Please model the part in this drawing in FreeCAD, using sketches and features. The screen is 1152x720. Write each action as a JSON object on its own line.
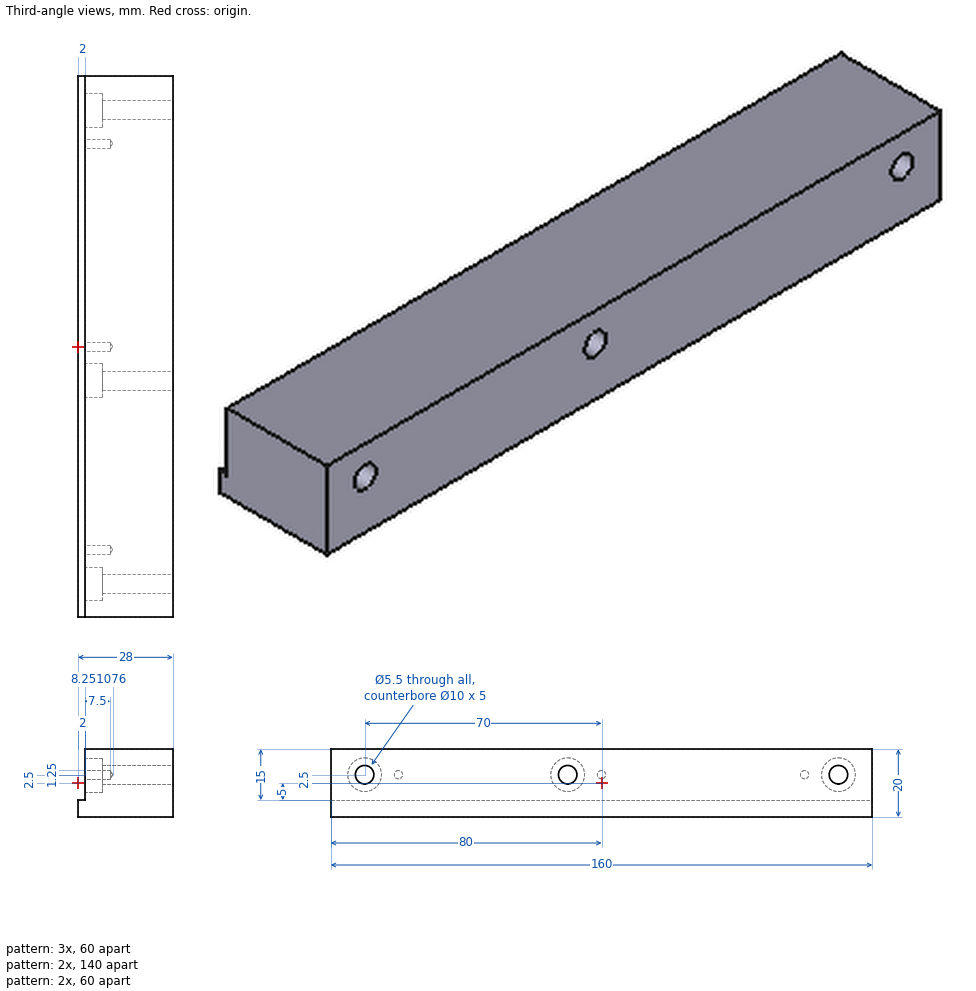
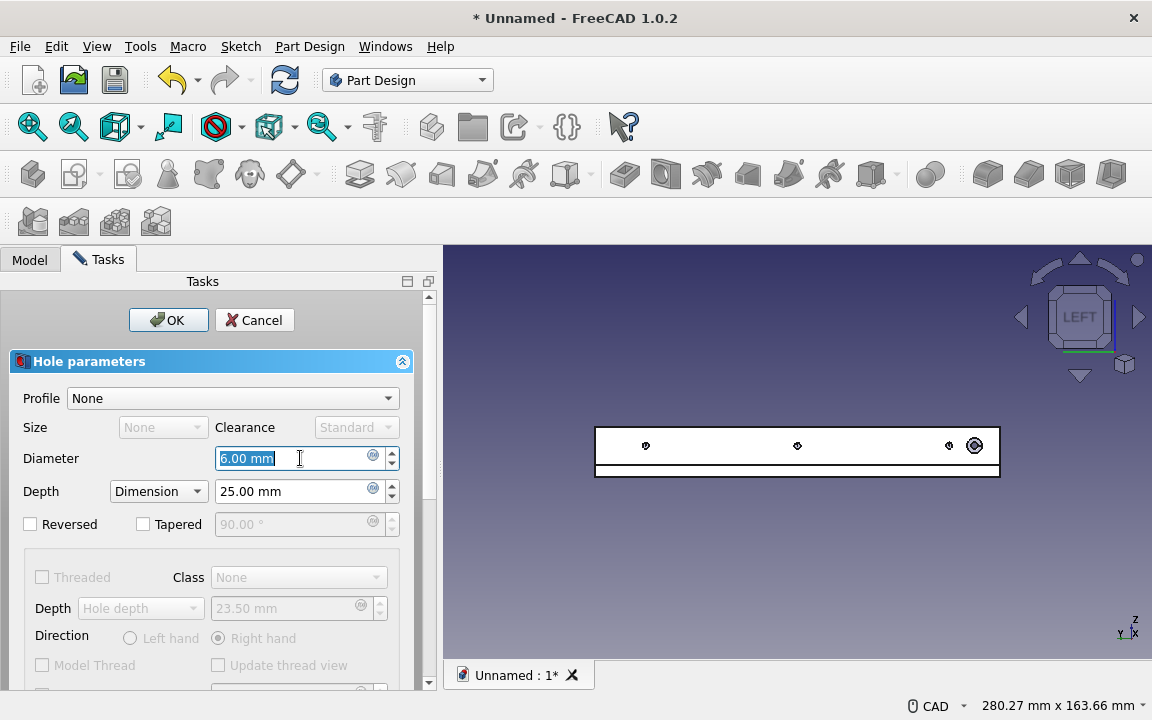
{"action": "type", "text": "5.5"}
{"action": "key", "text": "Tab"}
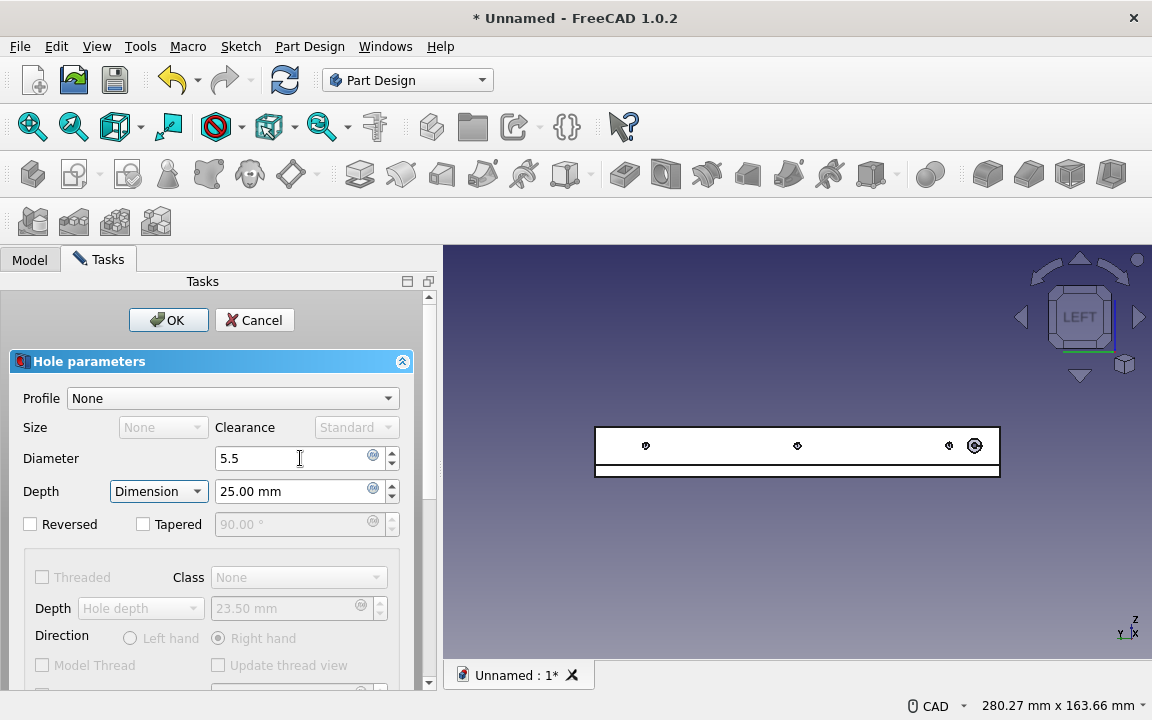
{"action": "left_click", "coordinate": [160, 492]}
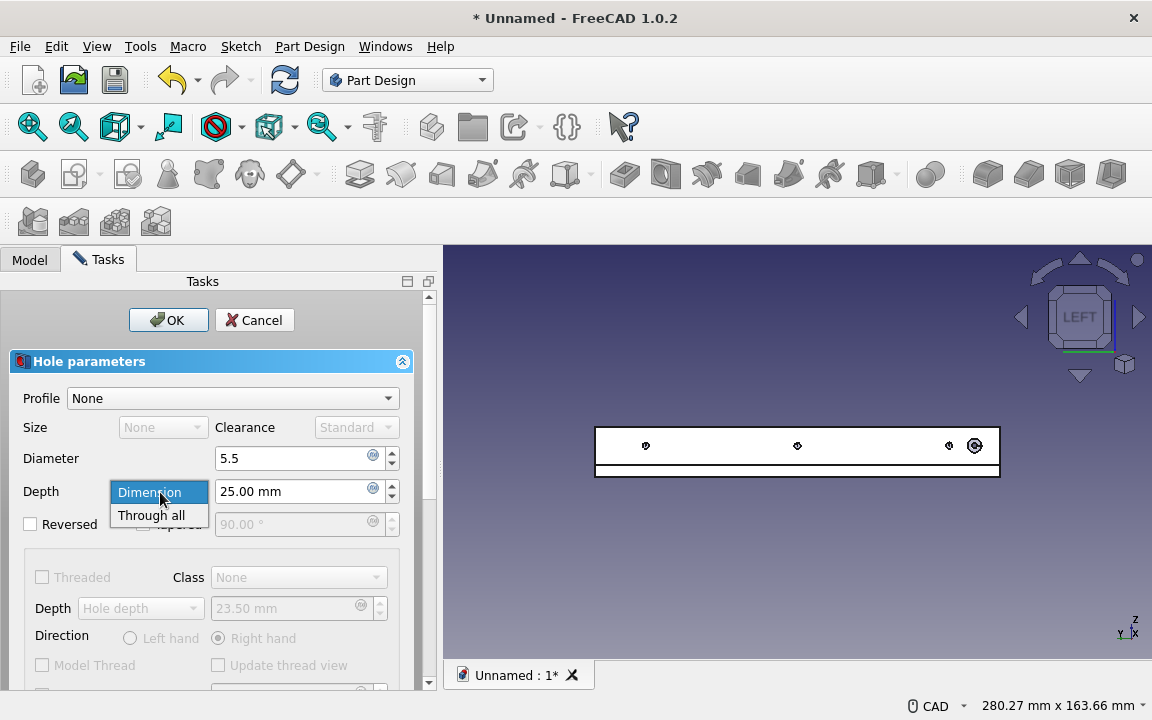
{"action": "left_click", "coordinate": [158, 516]}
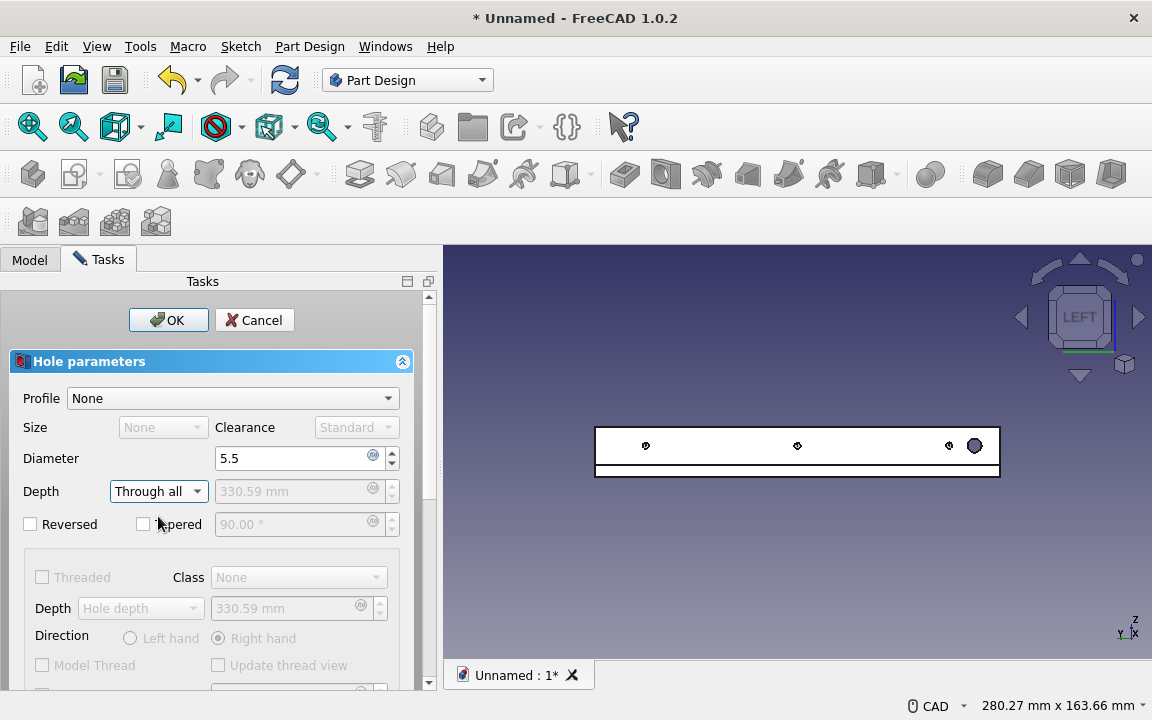
{"action": "scroll", "coordinate": [429, 490], "scroll_direction": "down", "scroll_amount": 3}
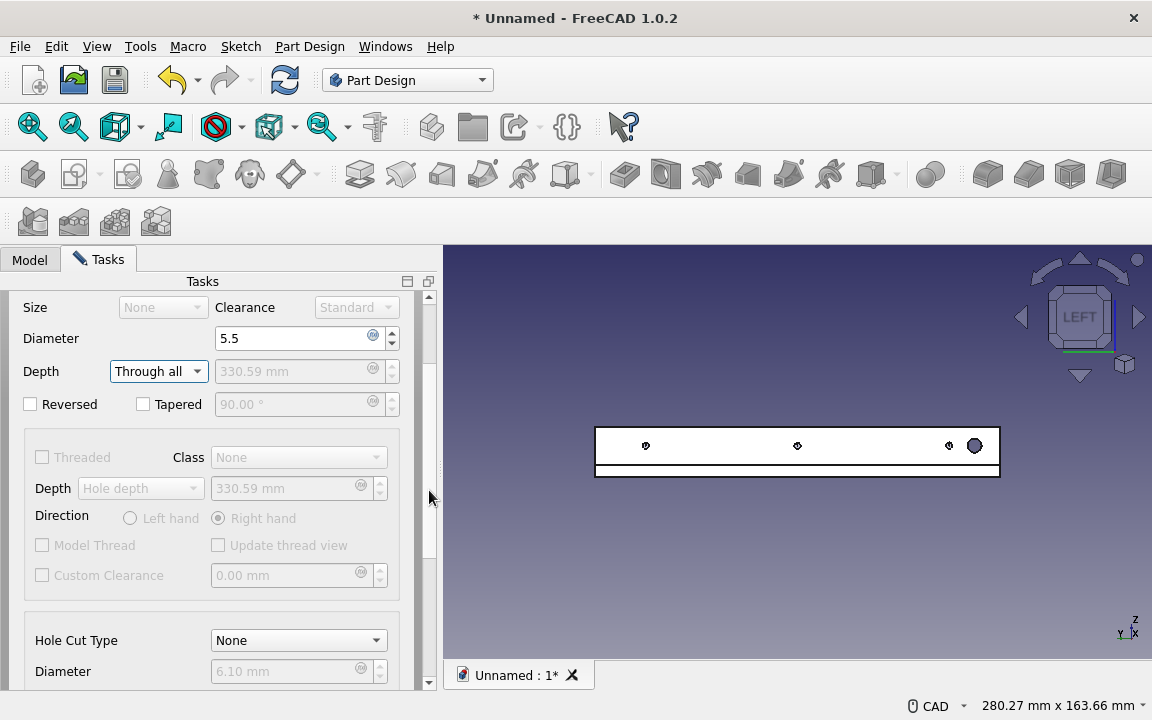
{"action": "left_click", "coordinate": [300, 580]}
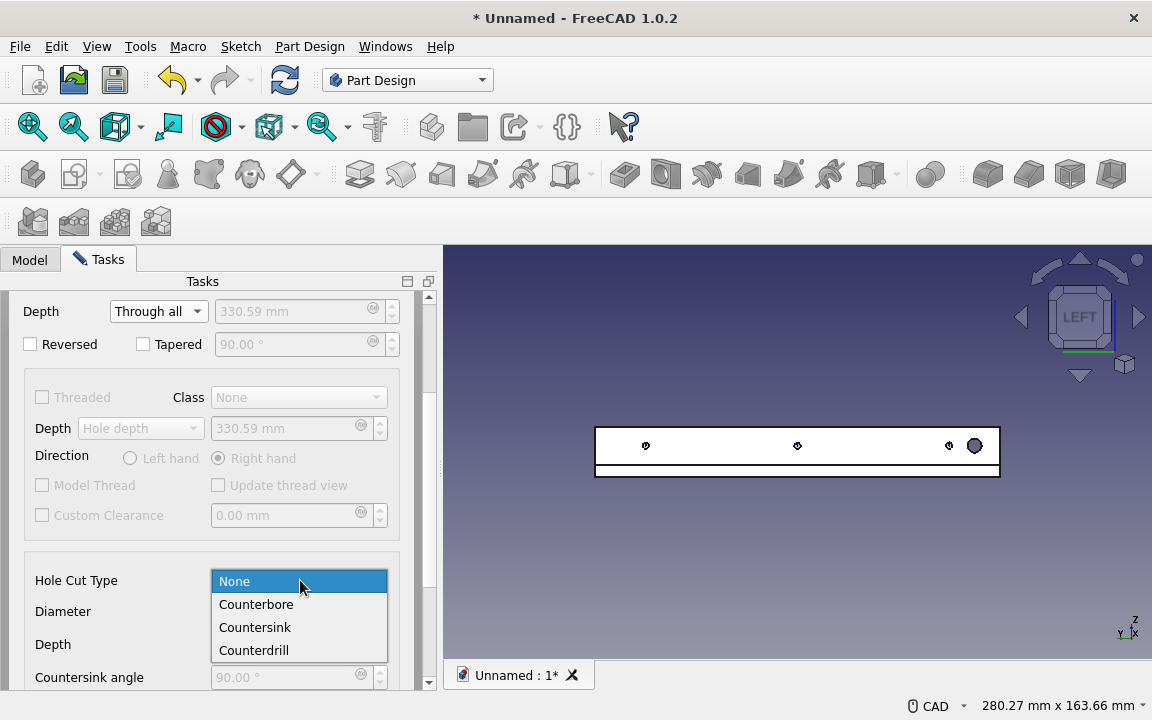
{"action": "left_click", "coordinate": [298, 604]}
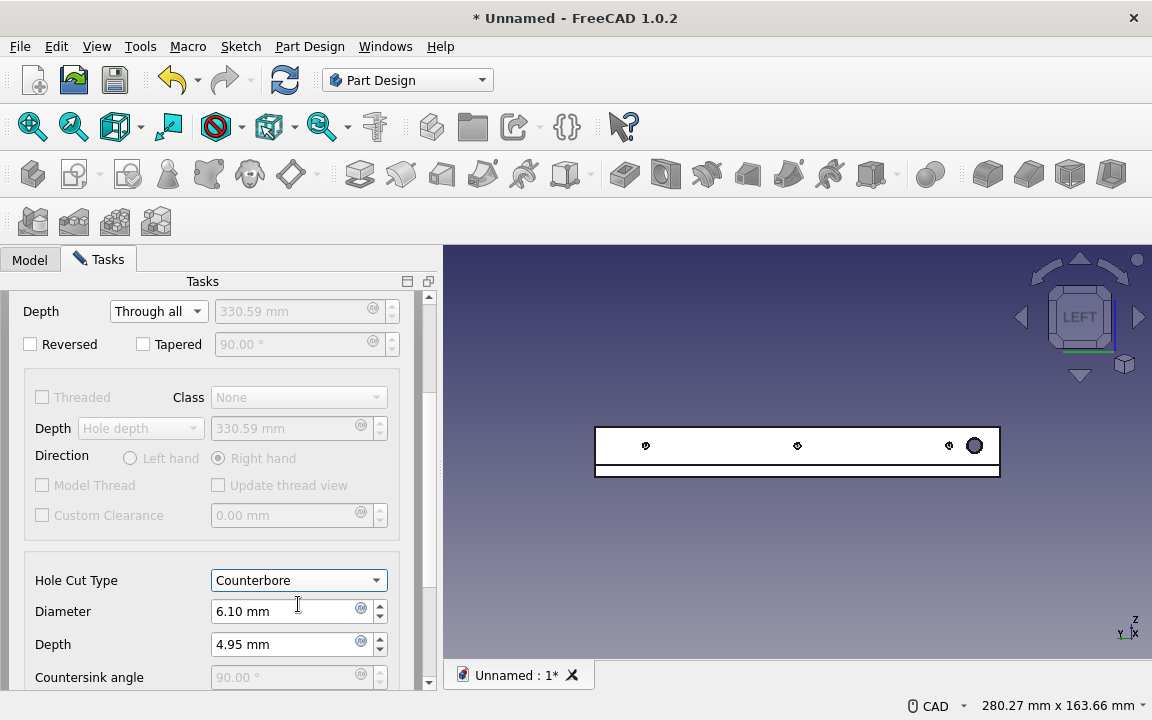
{"action": "triple_click", "coordinate": [292, 612]}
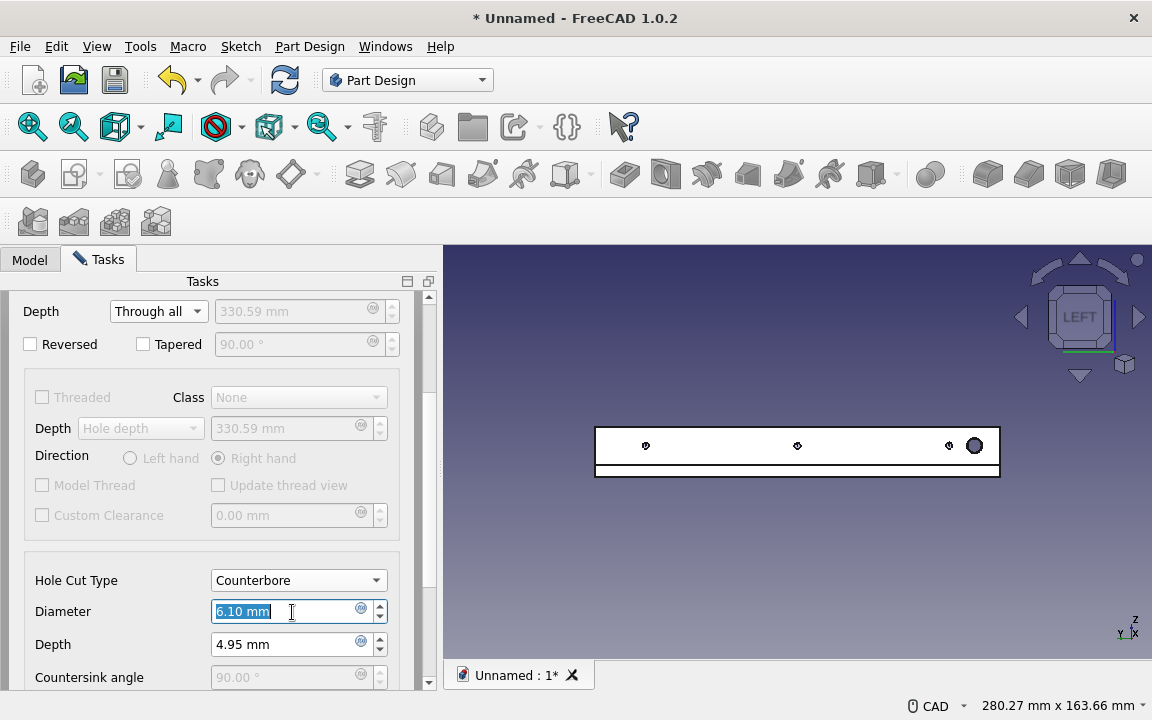
{"action": "type", "text": "10"}
{"action": "key", "text": "Tab"}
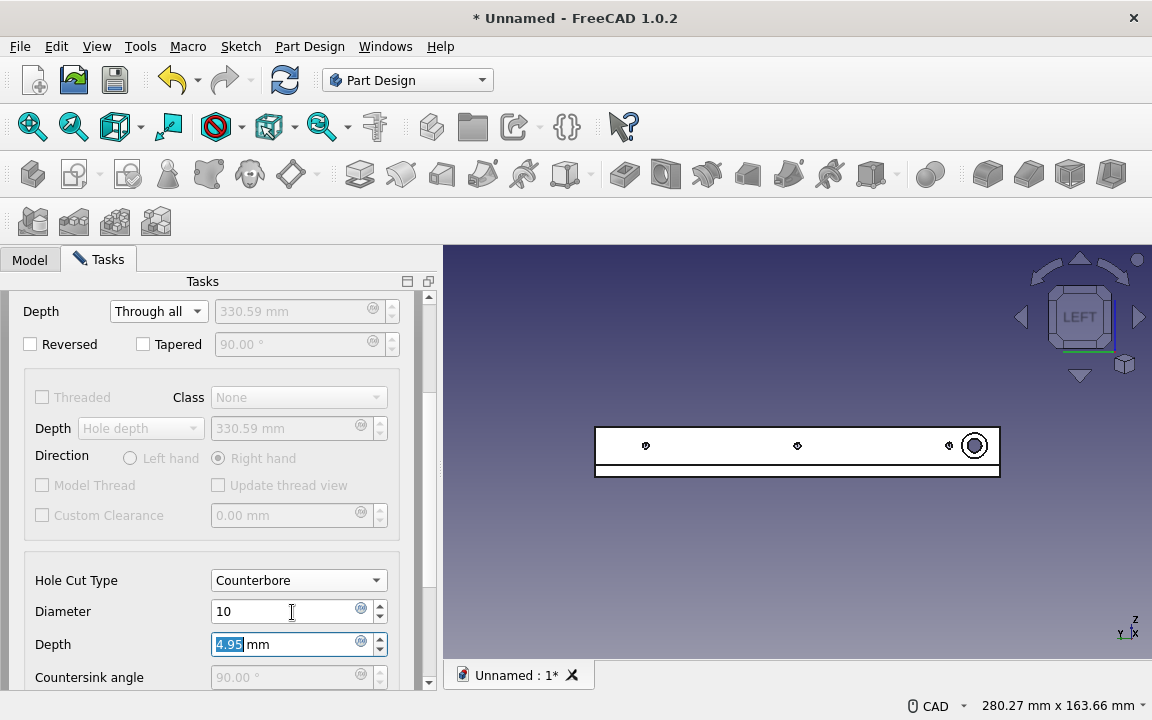
{"action": "type", "text": "5"}
{"action": "key", "text": "Tab"}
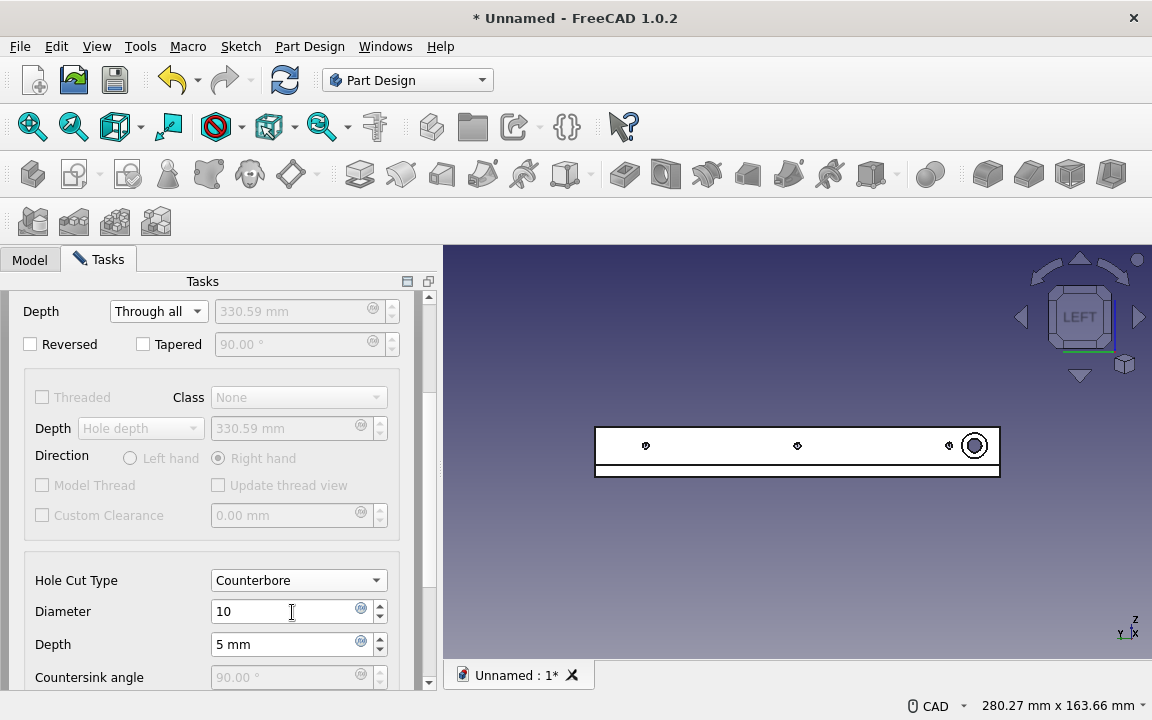
{"action": "scroll", "coordinate": [429, 490], "scroll_direction": "up", "scroll_amount": 4}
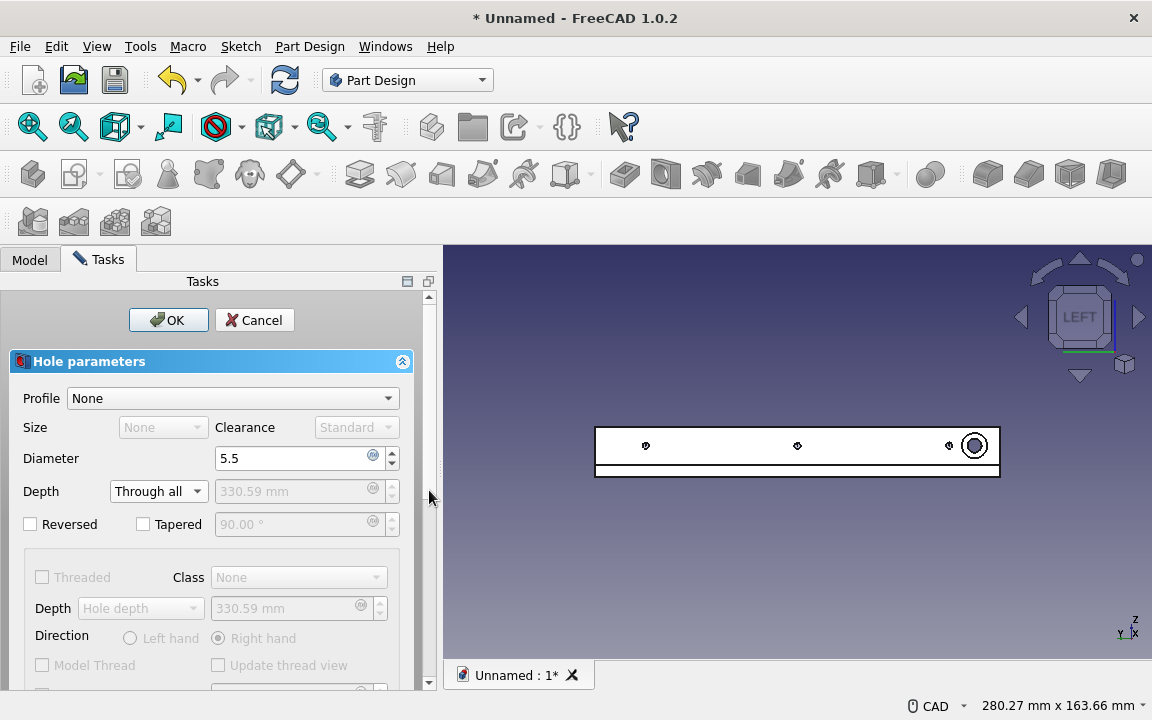
{"action": "left_click", "coordinate": [169, 320]}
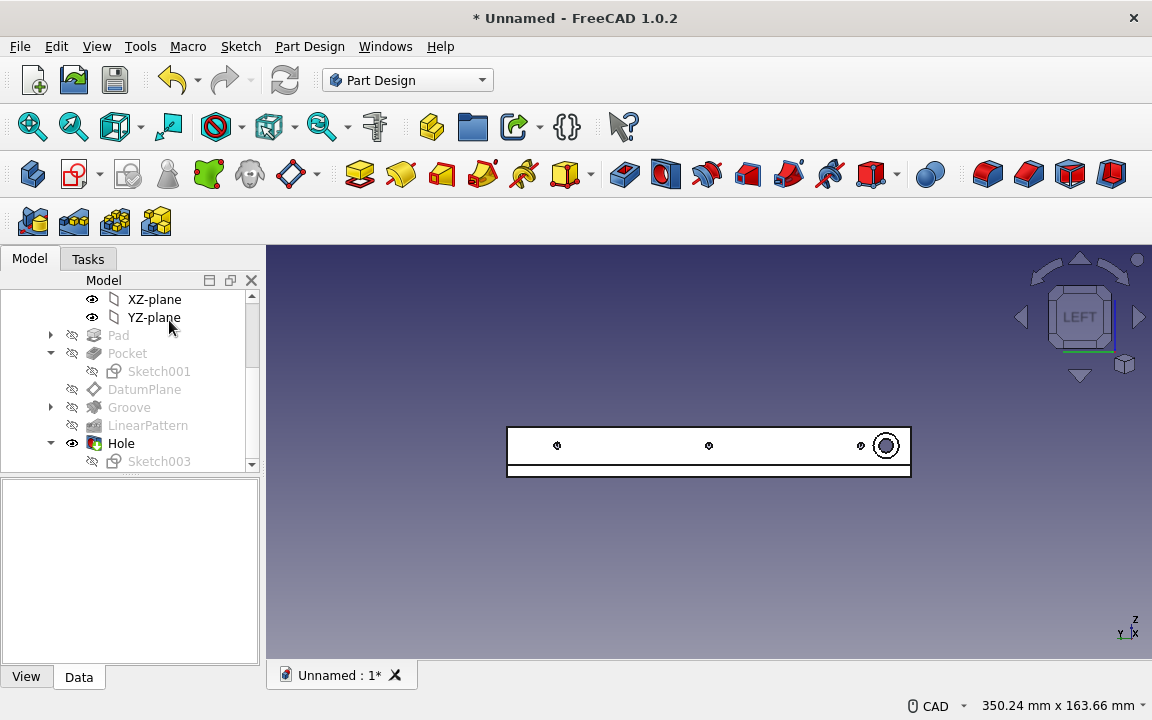
{"action": "left_click", "coordinate": [117, 443]}